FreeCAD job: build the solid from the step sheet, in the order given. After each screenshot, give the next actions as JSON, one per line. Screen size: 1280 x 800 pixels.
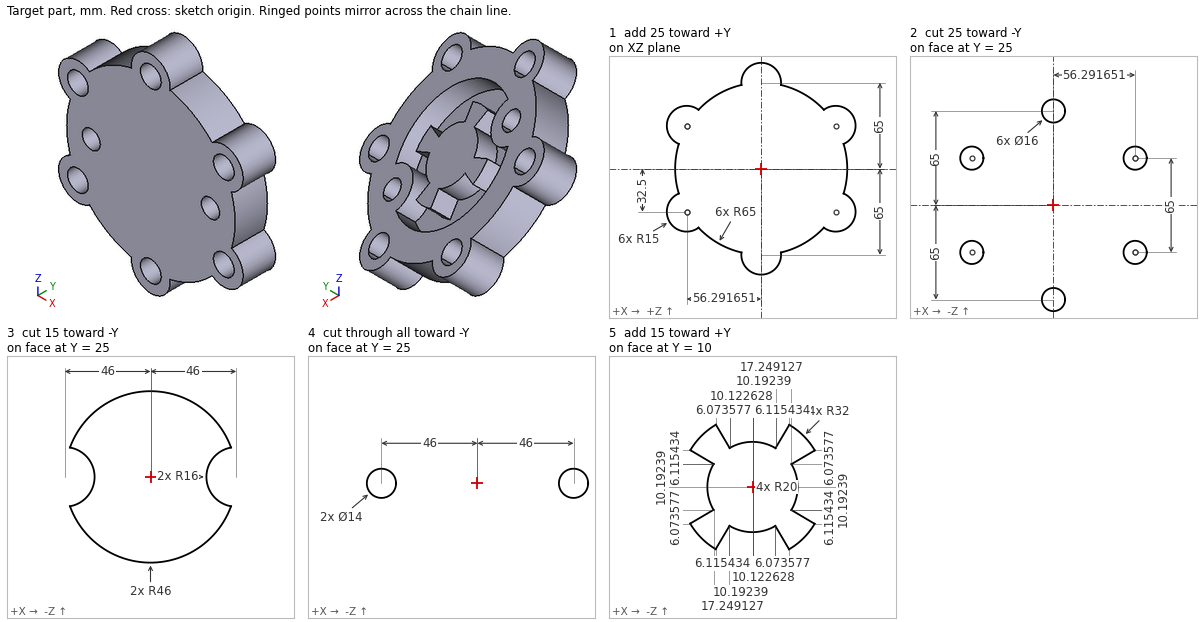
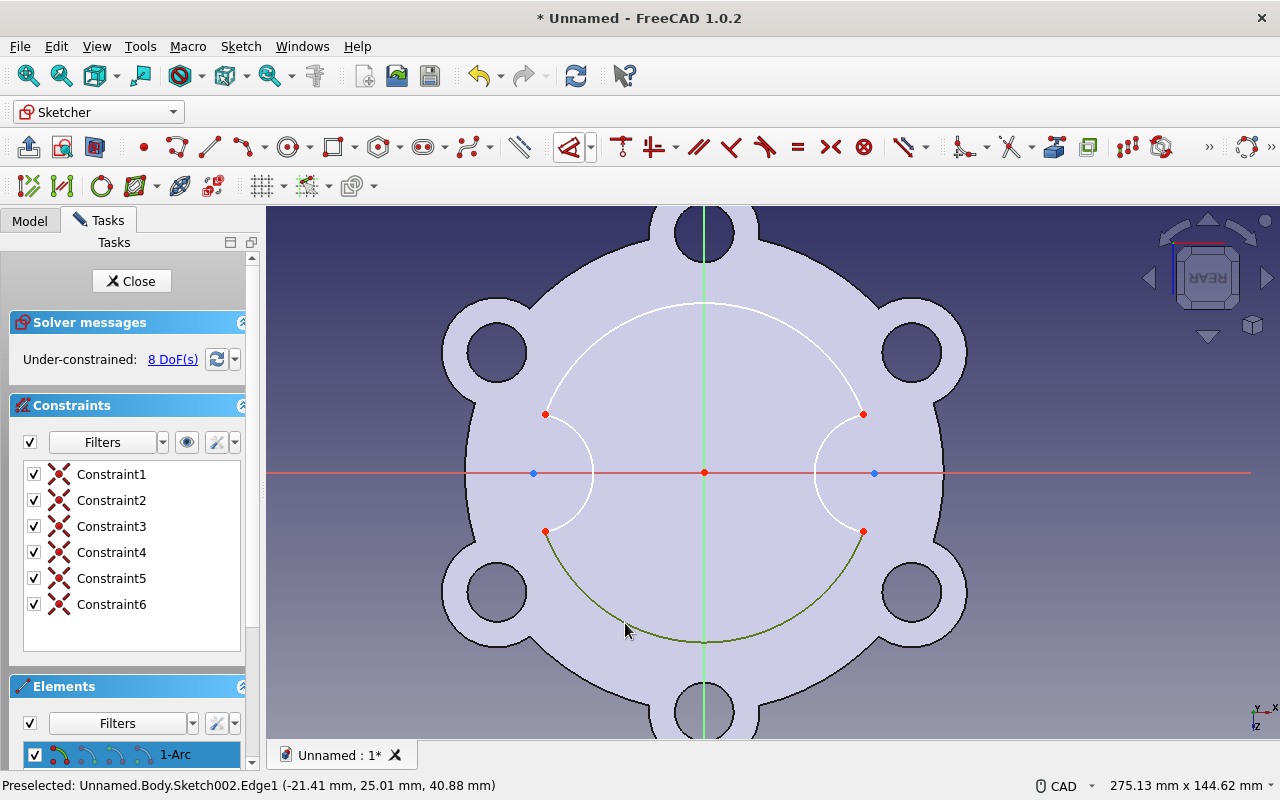
{"action": "left_click", "coordinate": [784, 323]}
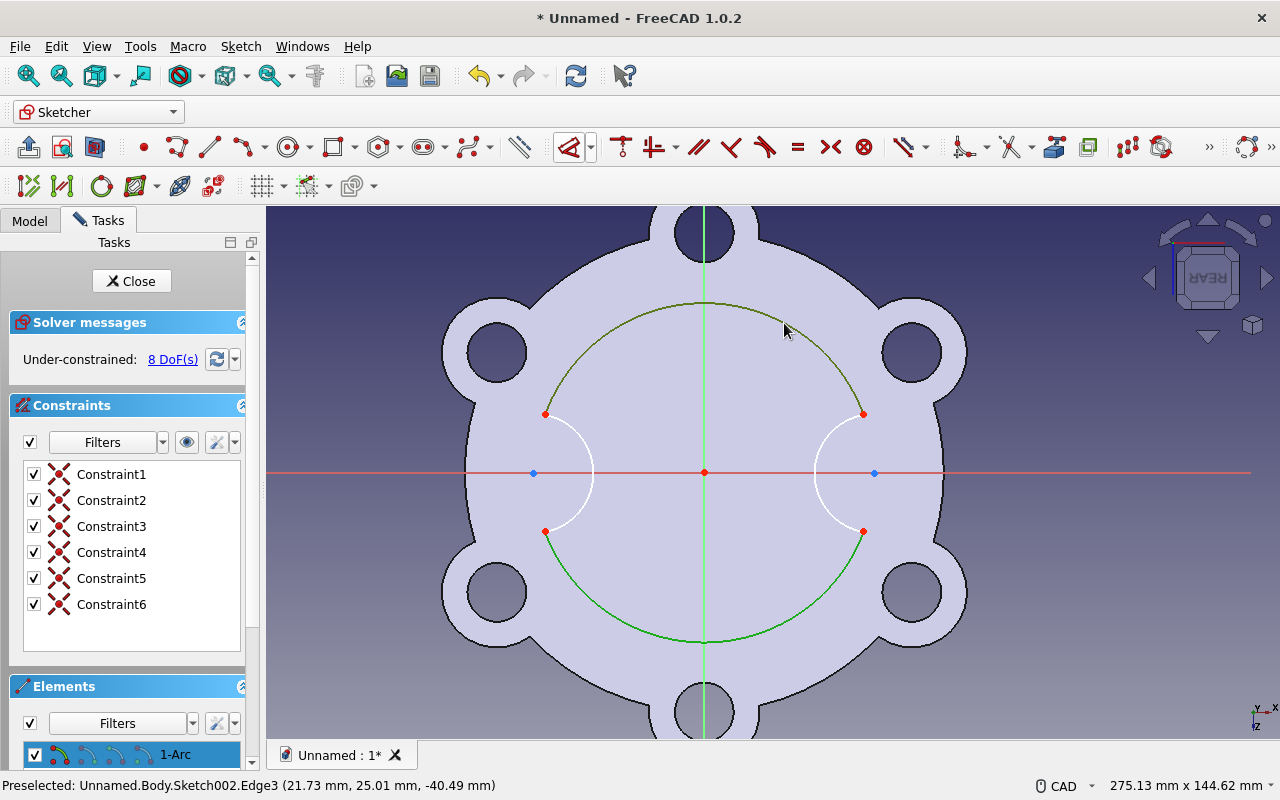
{"action": "left_click", "coordinate": [798, 148]}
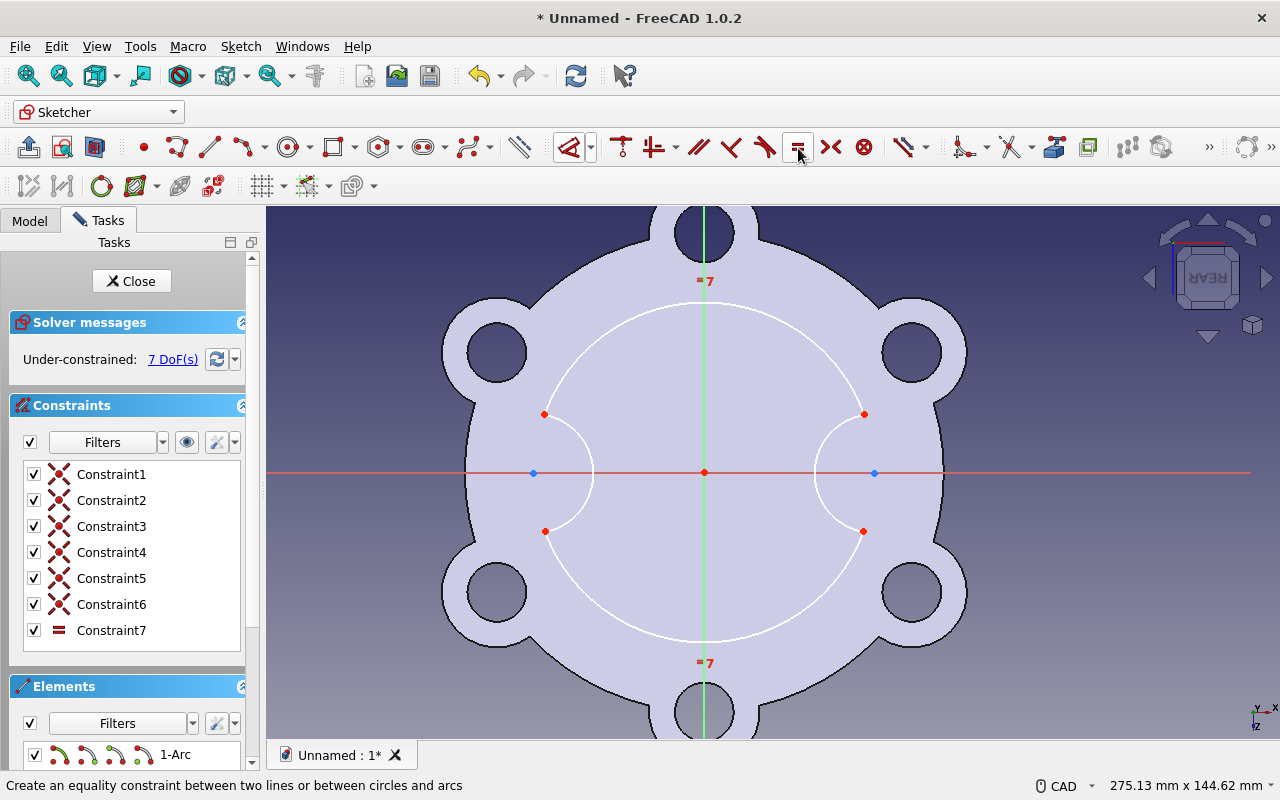
{"action": "left_click", "coordinate": [824, 442]}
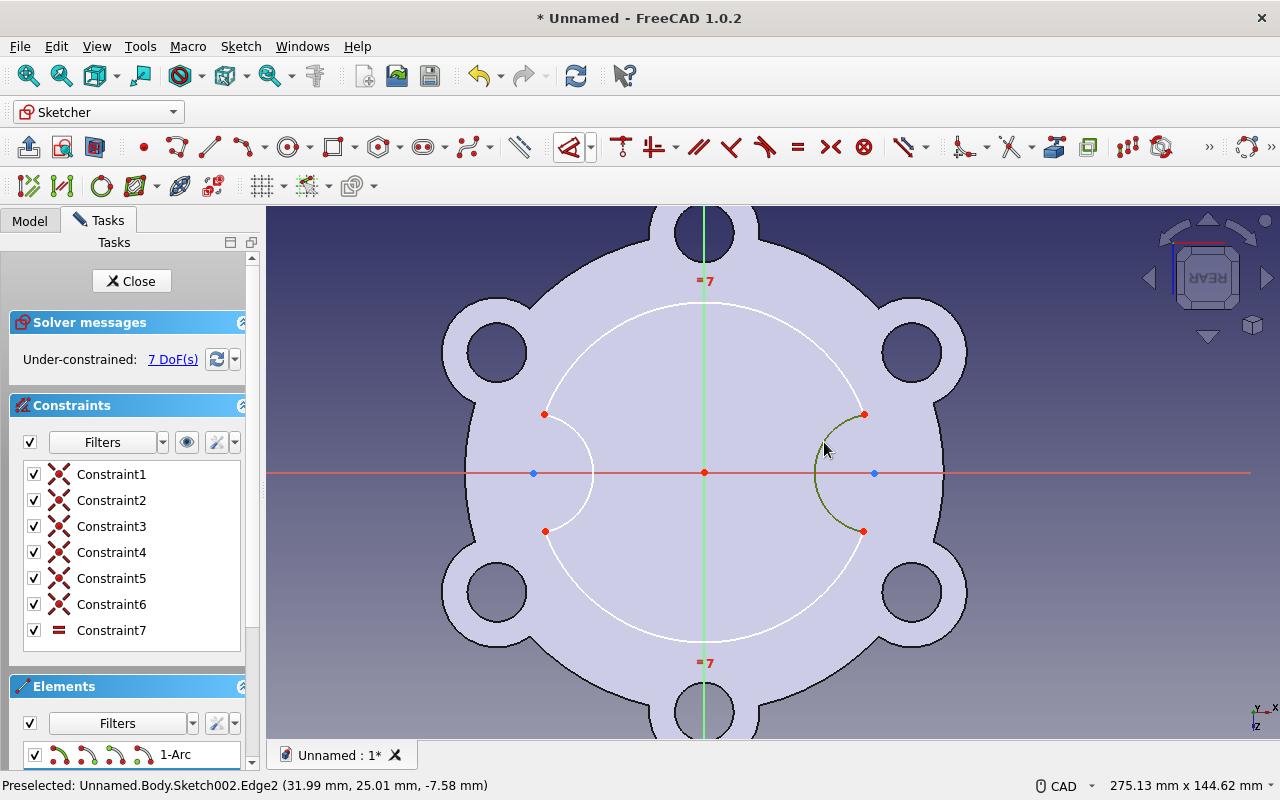
{"action": "left_click", "coordinate": [585, 505]}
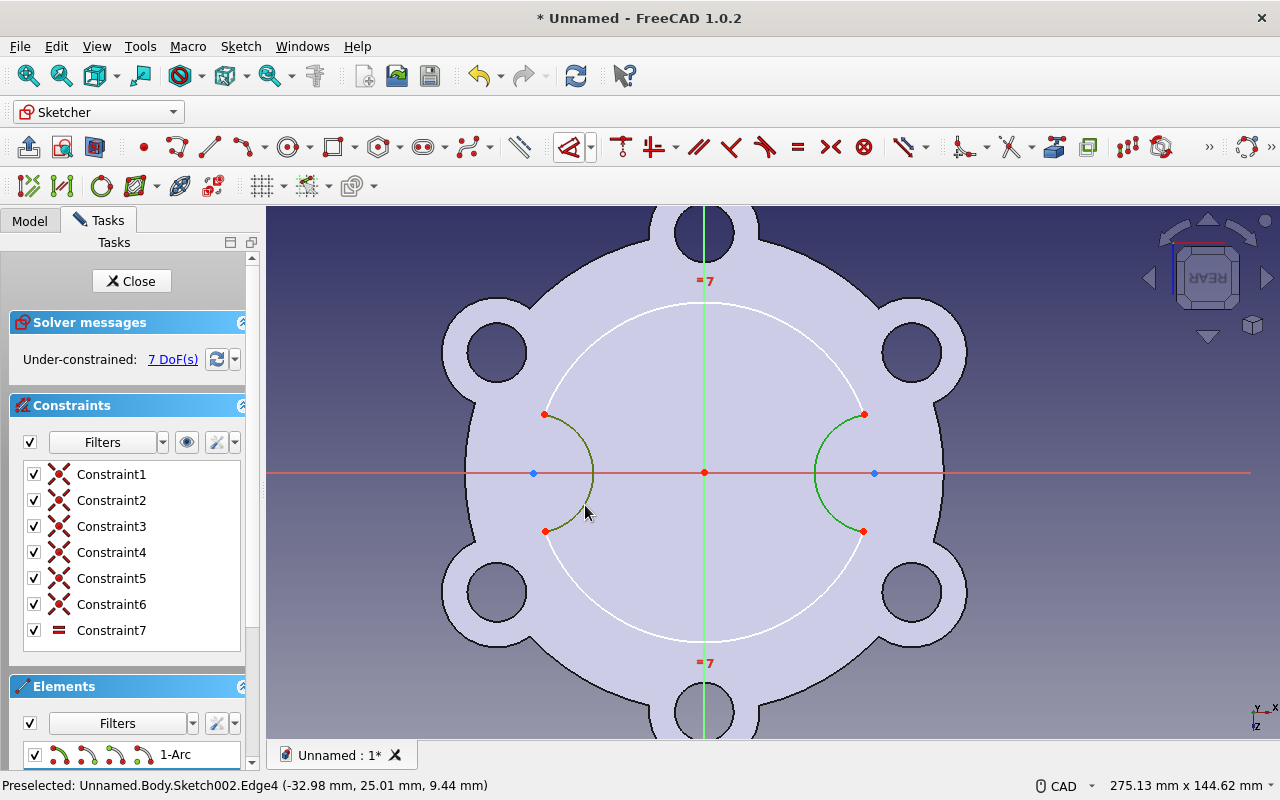
{"action": "left_click", "coordinate": [798, 148]}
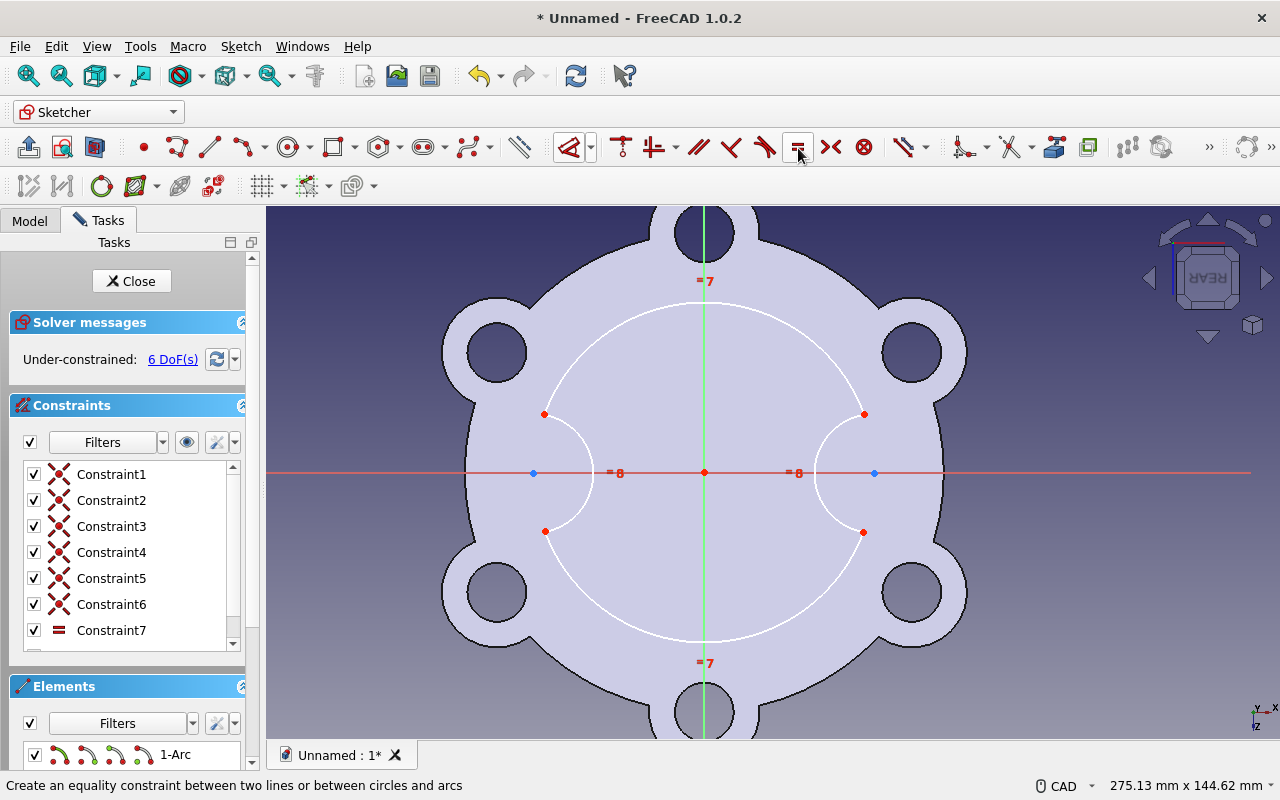
{"action": "left_click", "coordinate": [874, 474]}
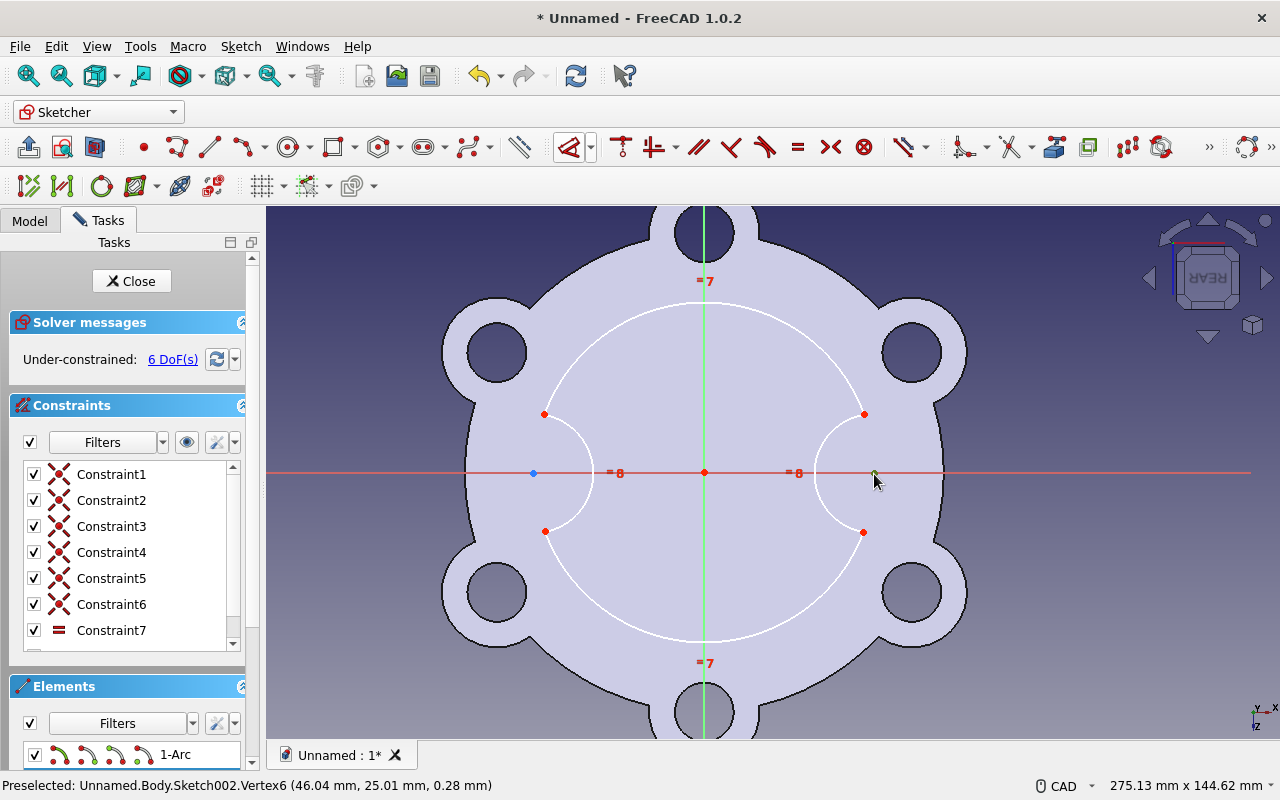
{"action": "left_click", "coordinate": [353, 472]}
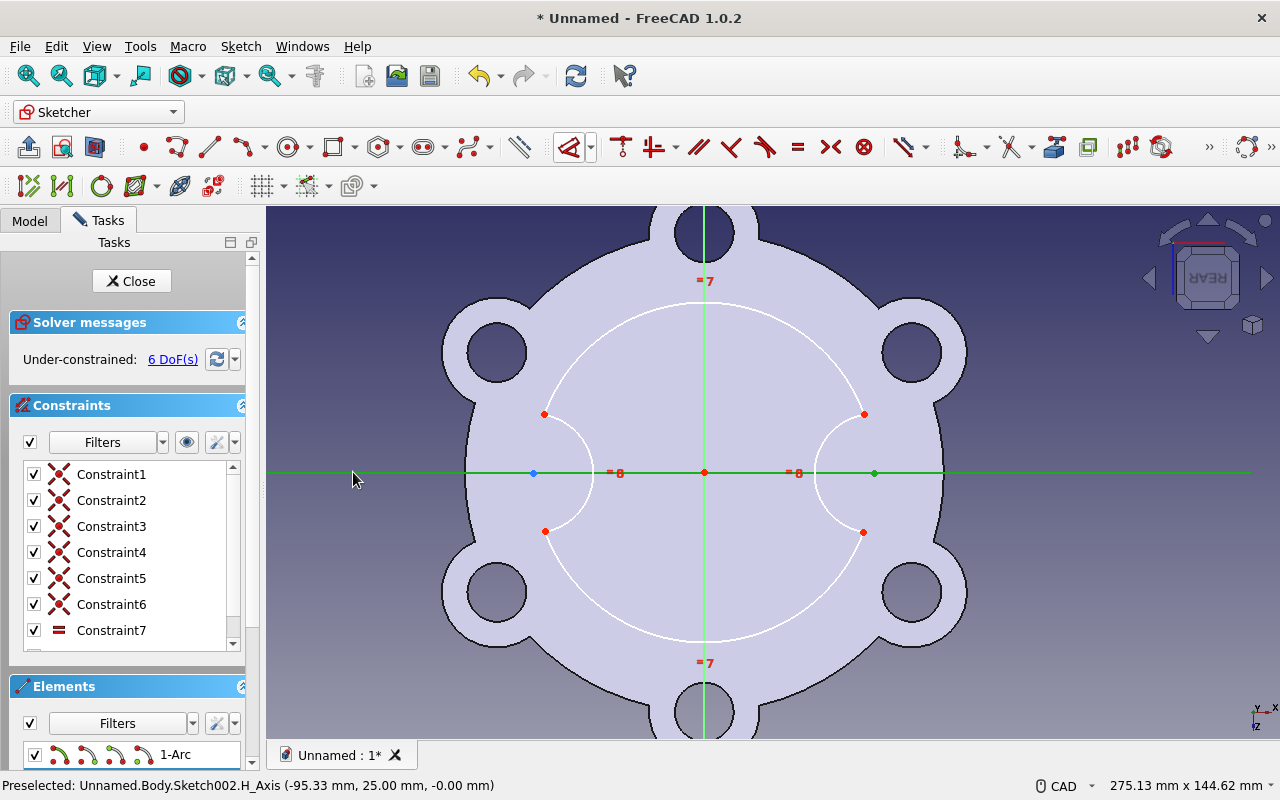
{"action": "left_click", "coordinate": [621, 148]}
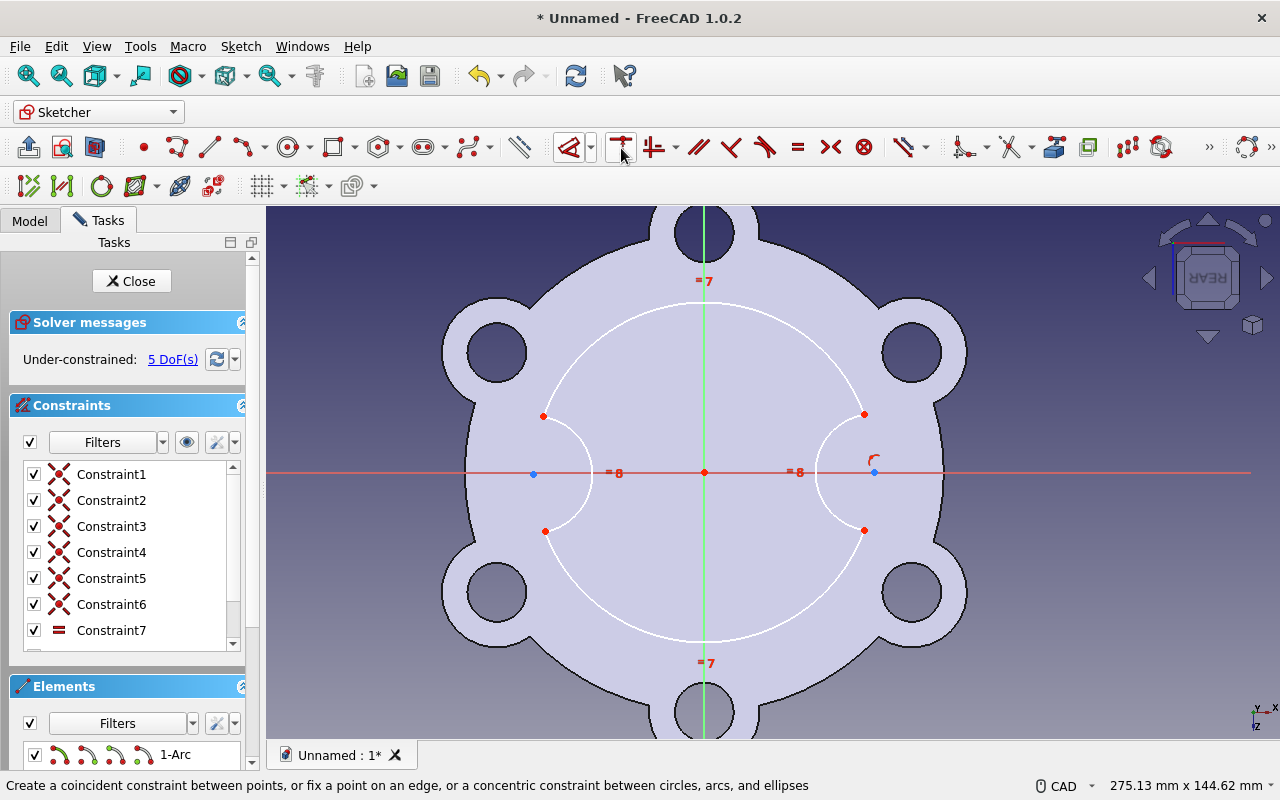
{"action": "left_click", "coordinate": [534, 475]}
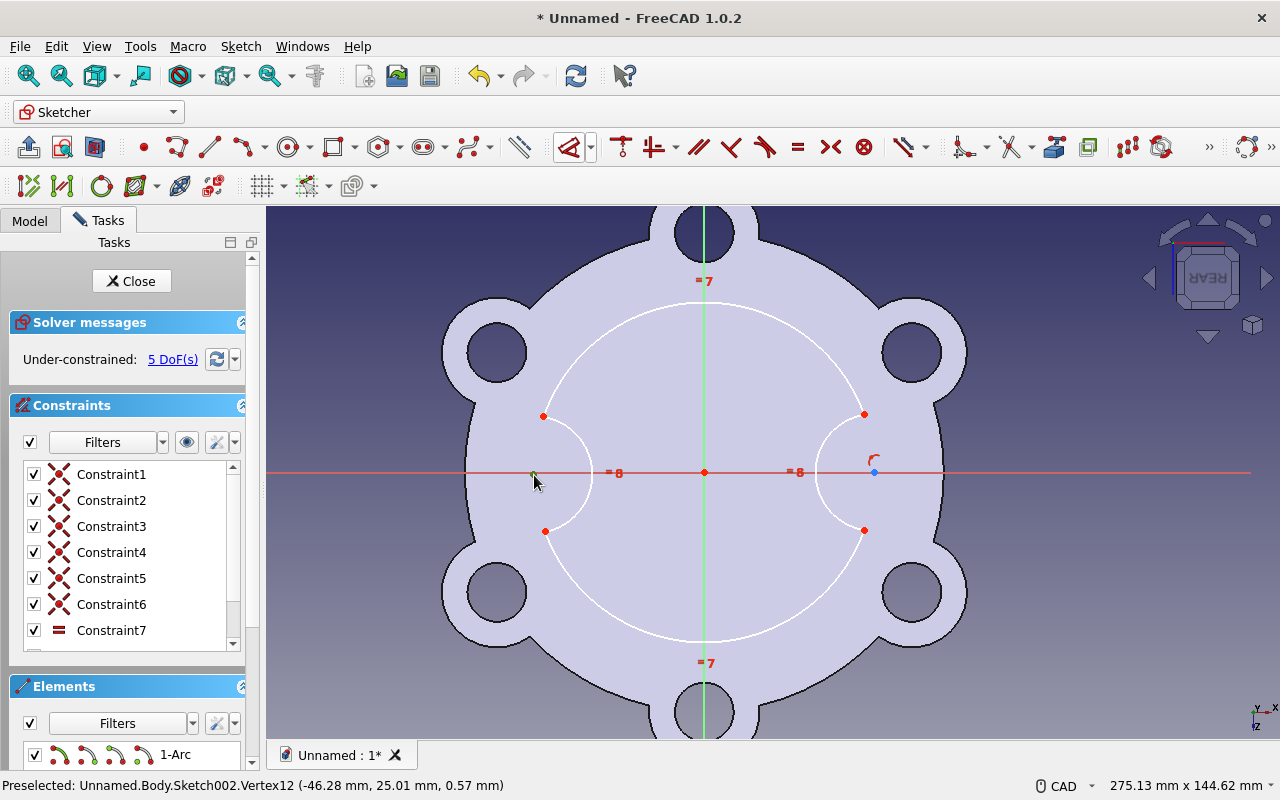
{"action": "left_click", "coordinate": [353, 472]}